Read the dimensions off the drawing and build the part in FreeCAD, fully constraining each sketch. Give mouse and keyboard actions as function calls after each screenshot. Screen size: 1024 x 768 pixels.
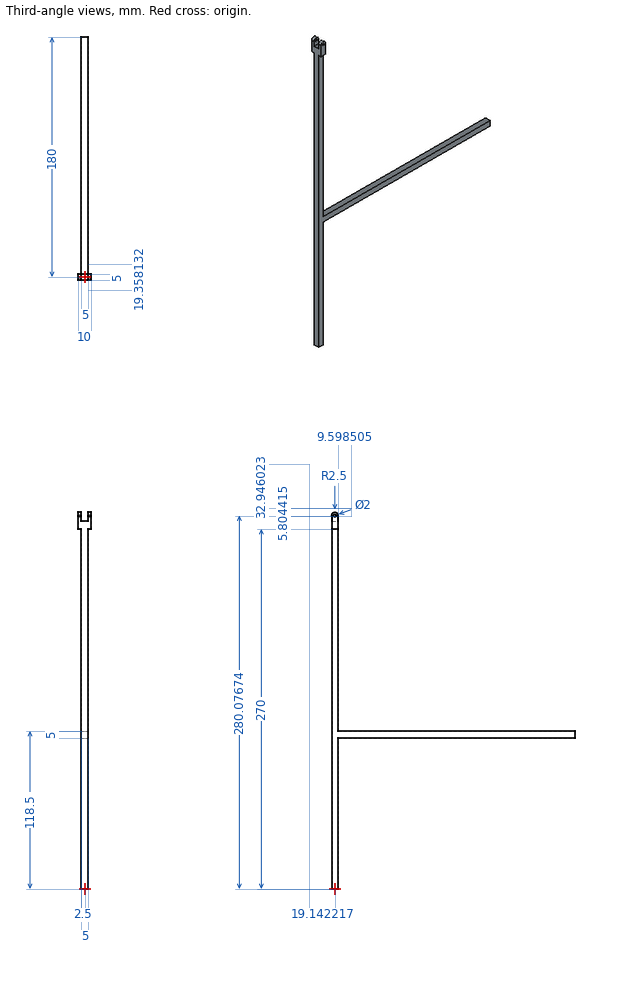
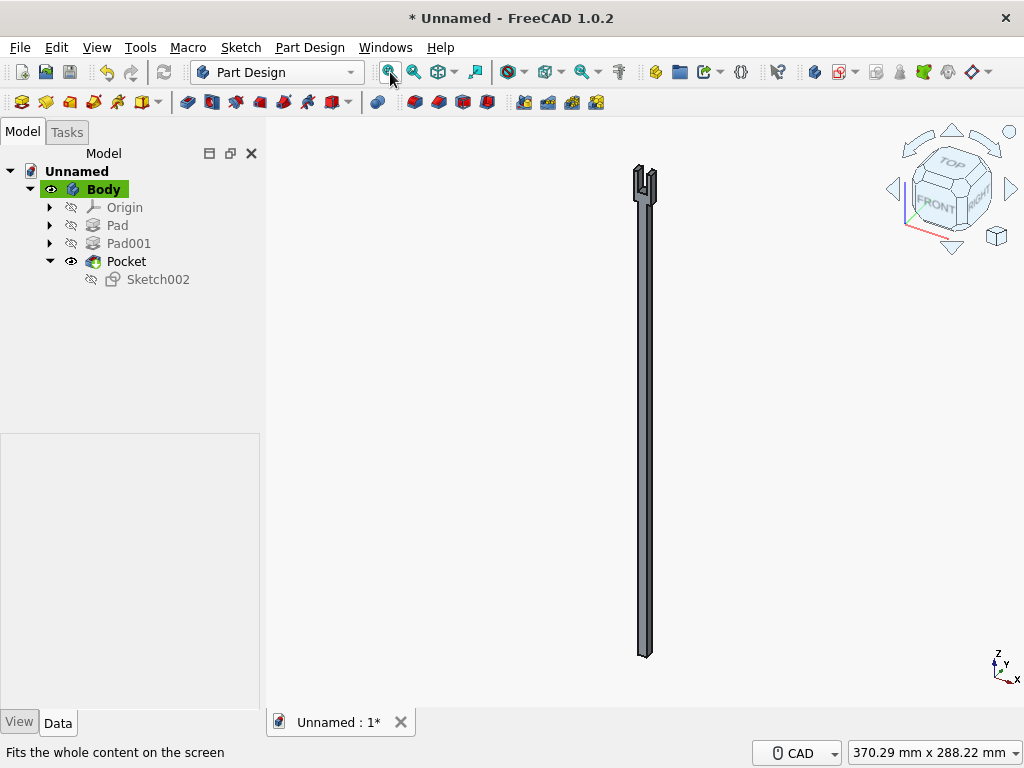
key(0)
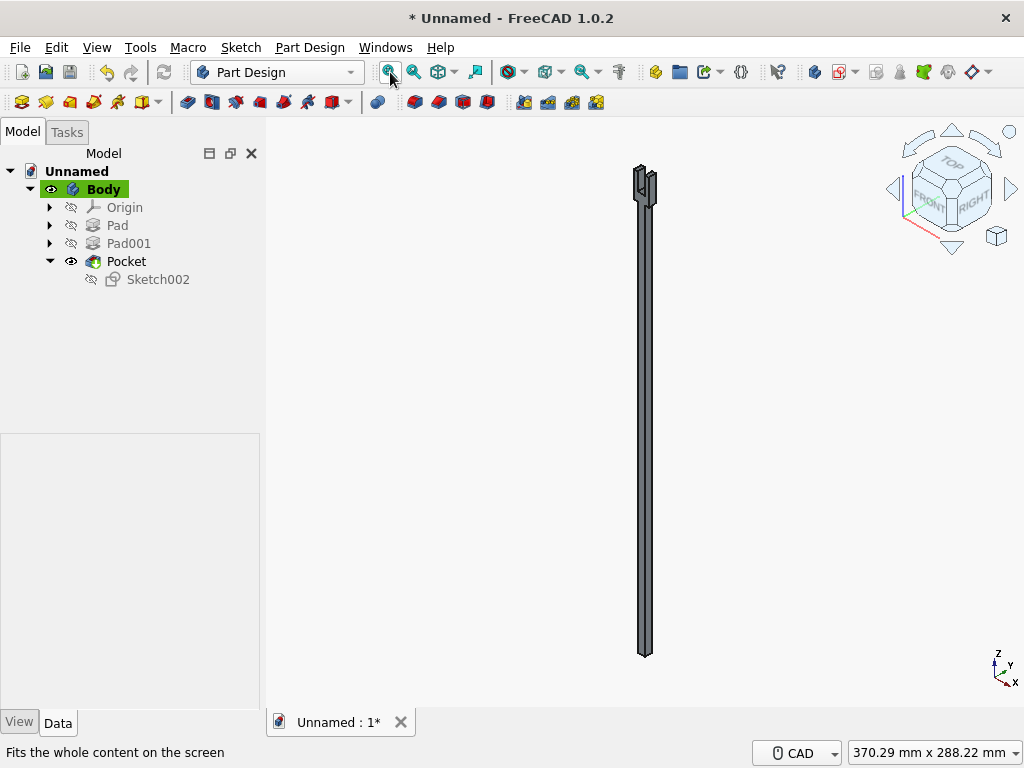
scroll(652, 181, up, 5)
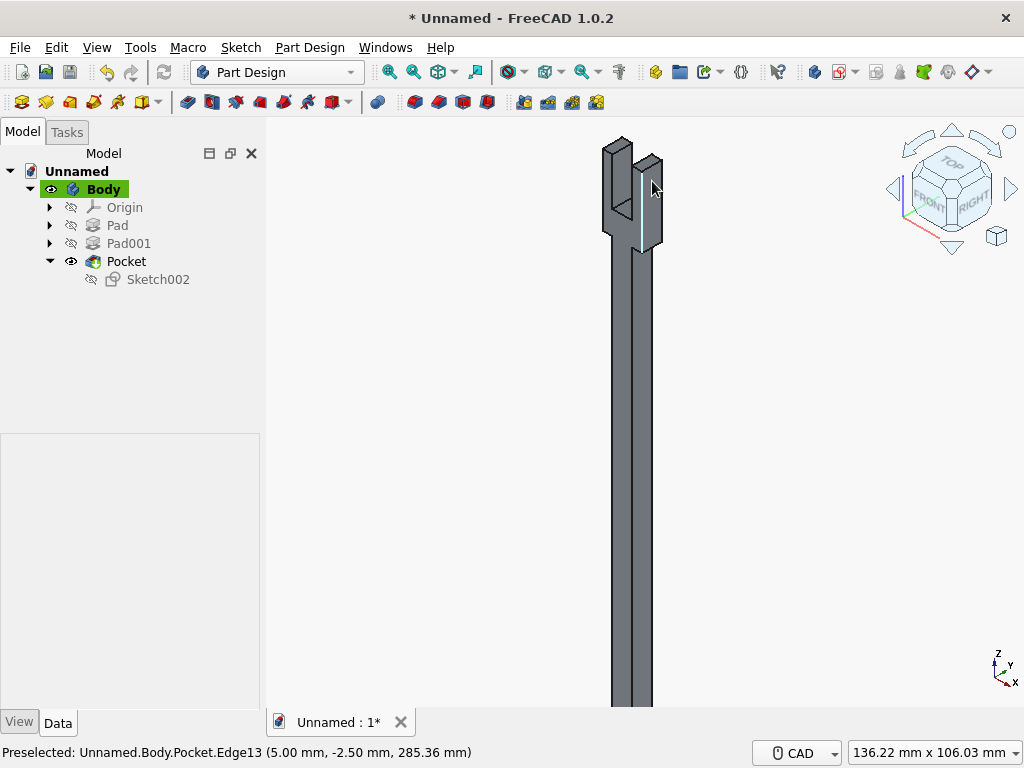
click(652, 182)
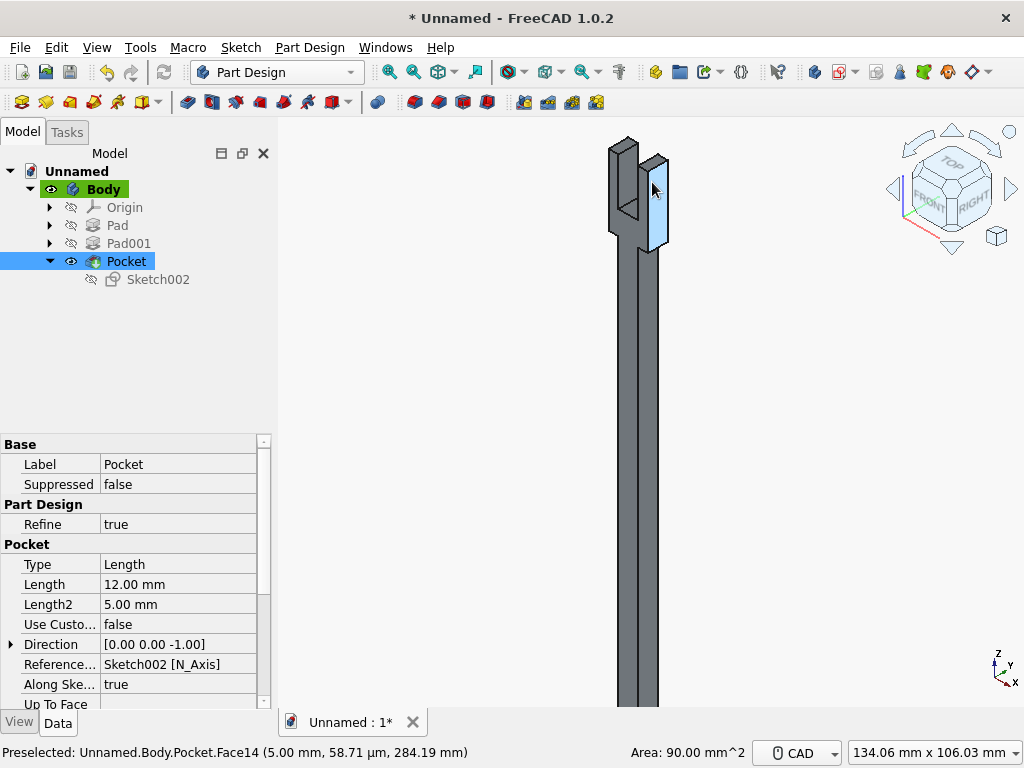
click(840, 72)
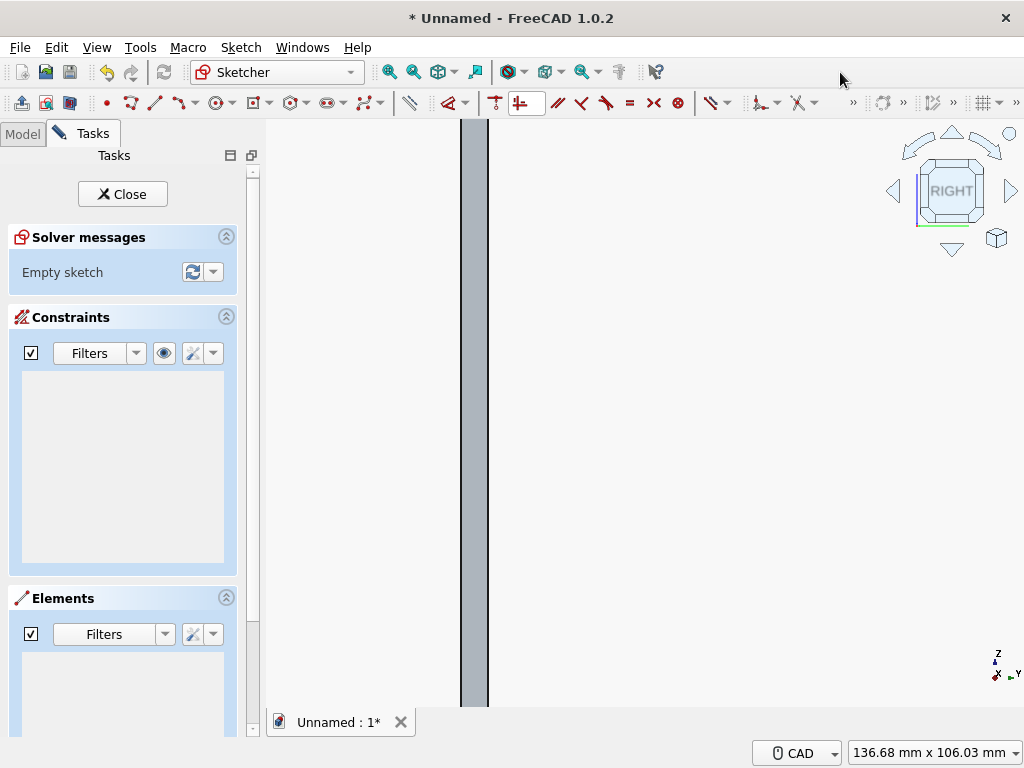
scroll(576, 413, down, 5)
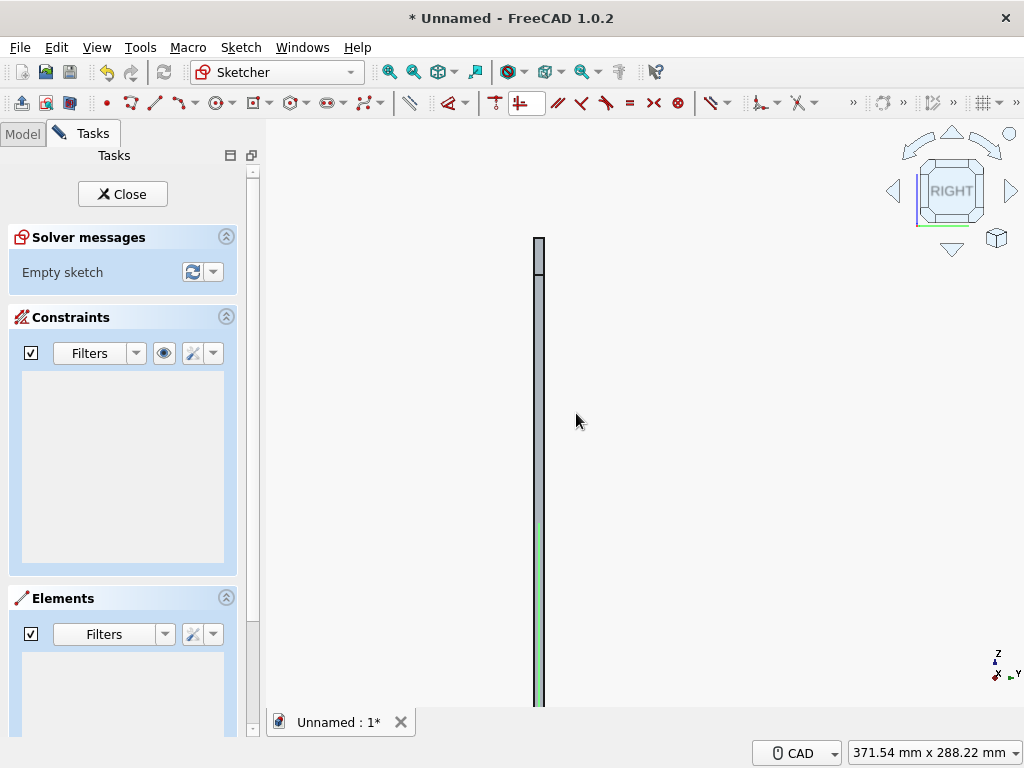
scroll(520, 166, up, 8)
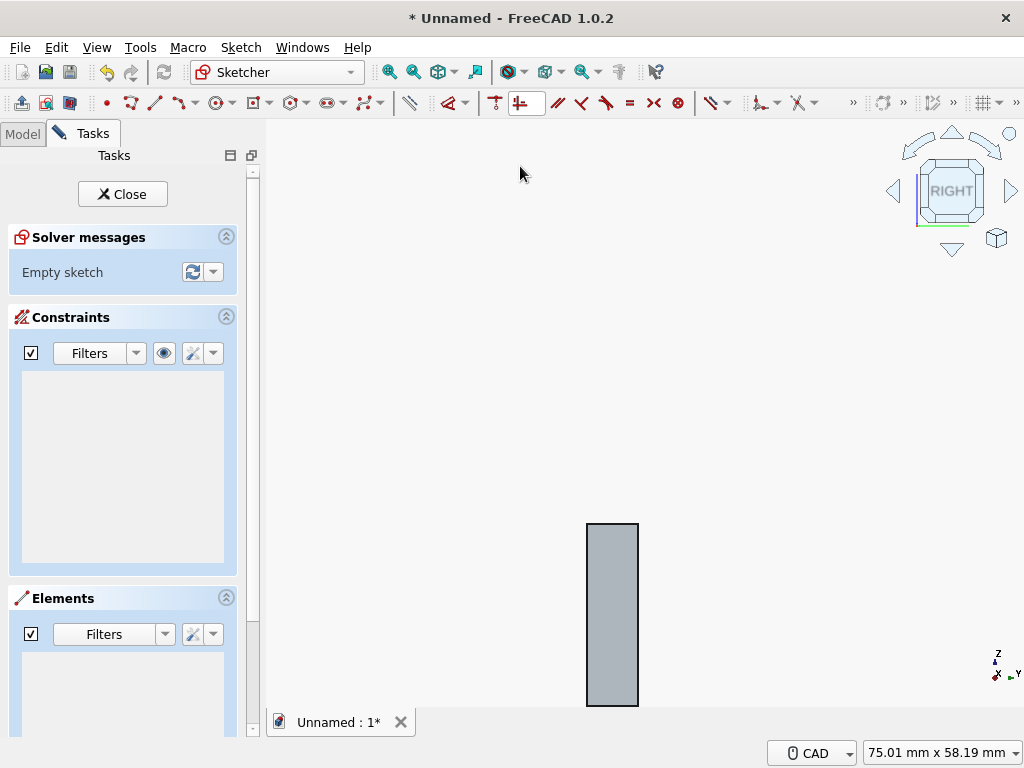
click(132, 104)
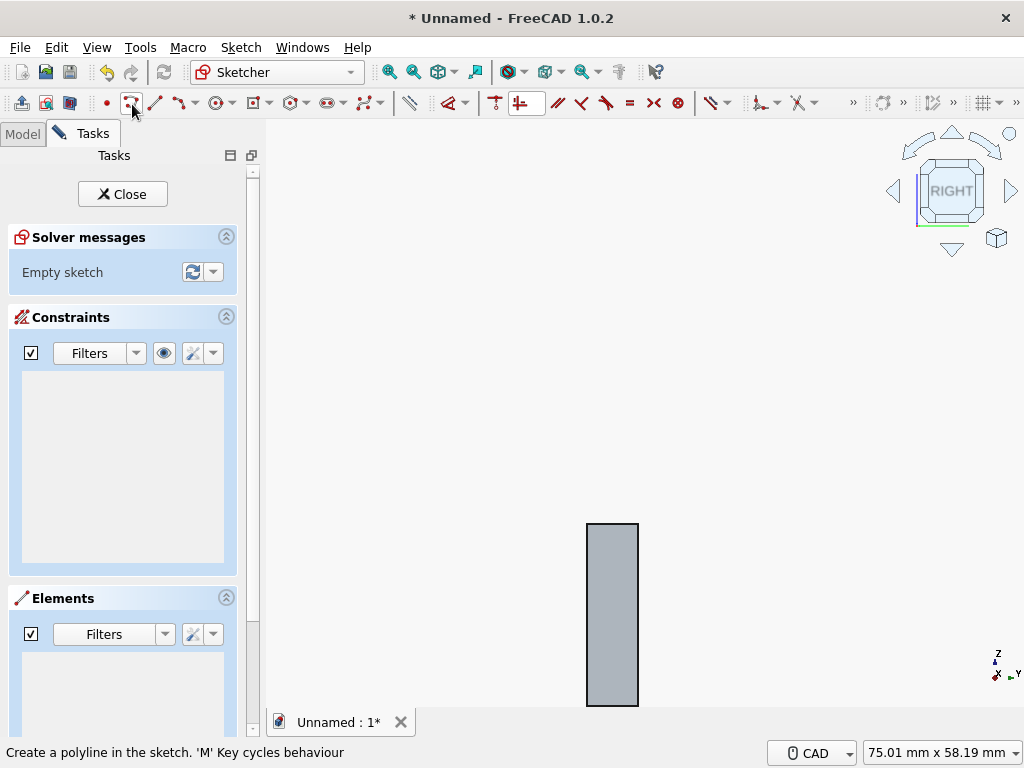
click(638, 604)
click(735, 604)
click(735, 545)
click(419, 212)
click(587, 604)
right_click(587, 604)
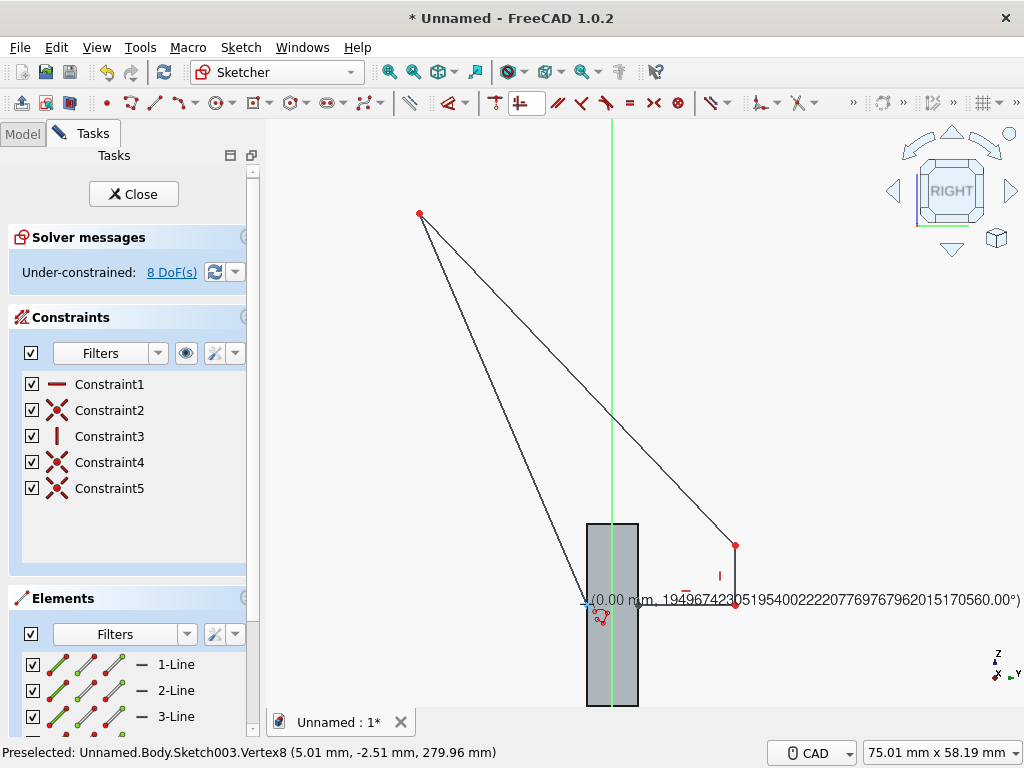
click(180, 104)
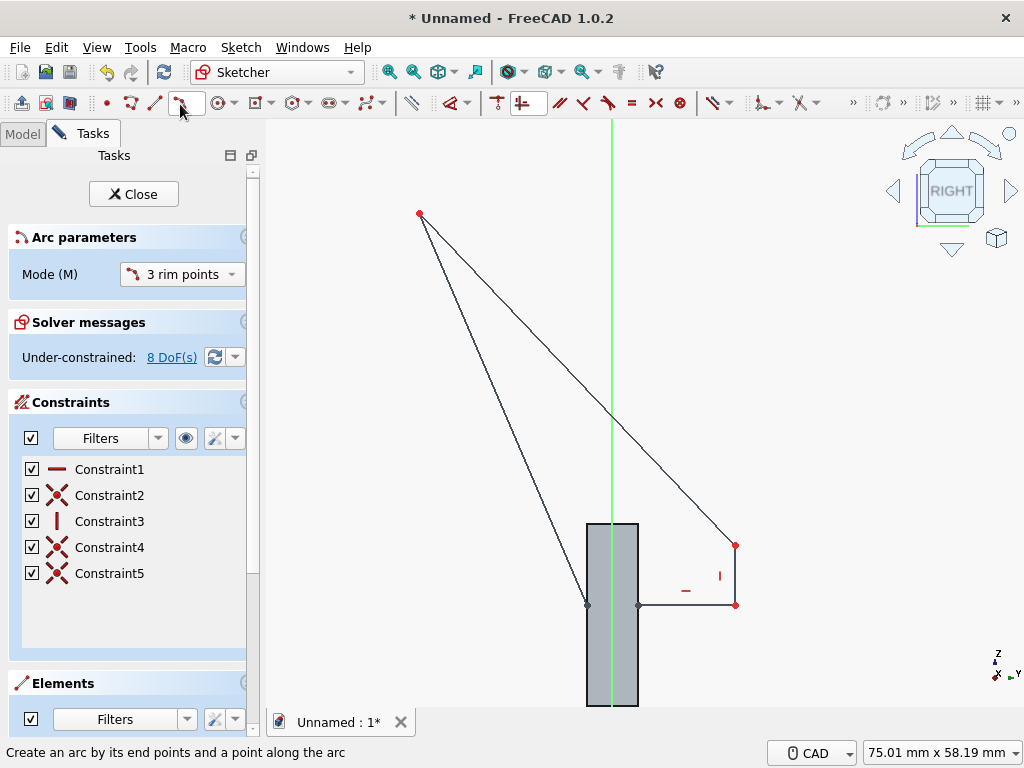
click(587, 605)
click(638, 605)
click(627, 583)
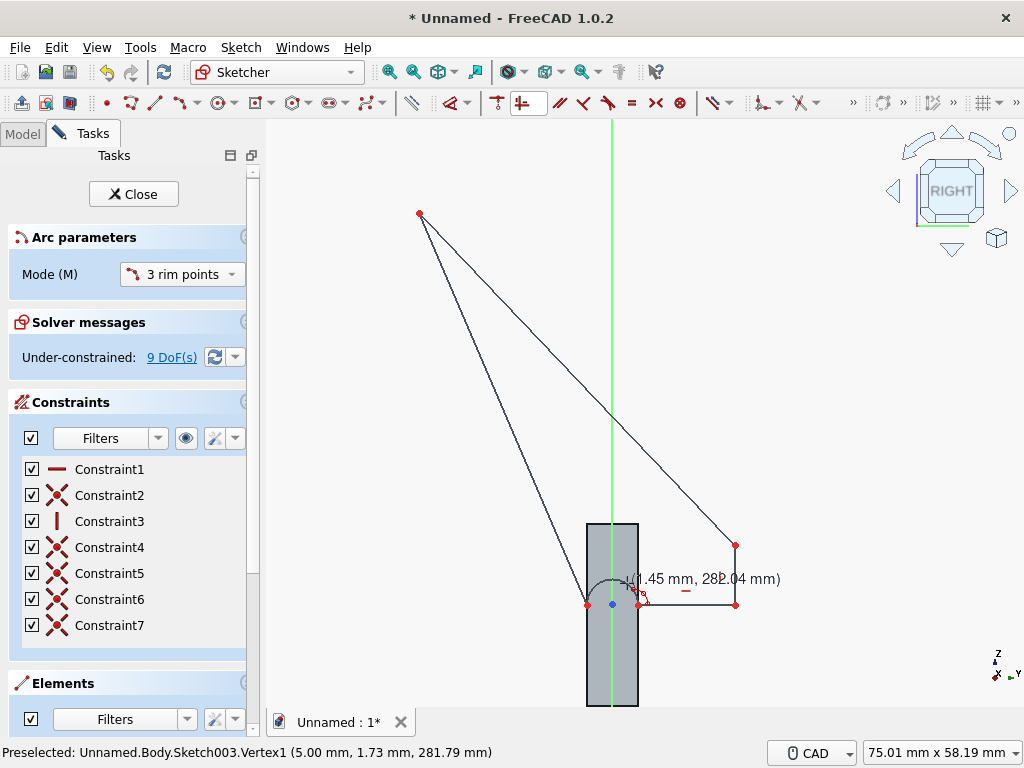
click(218, 104)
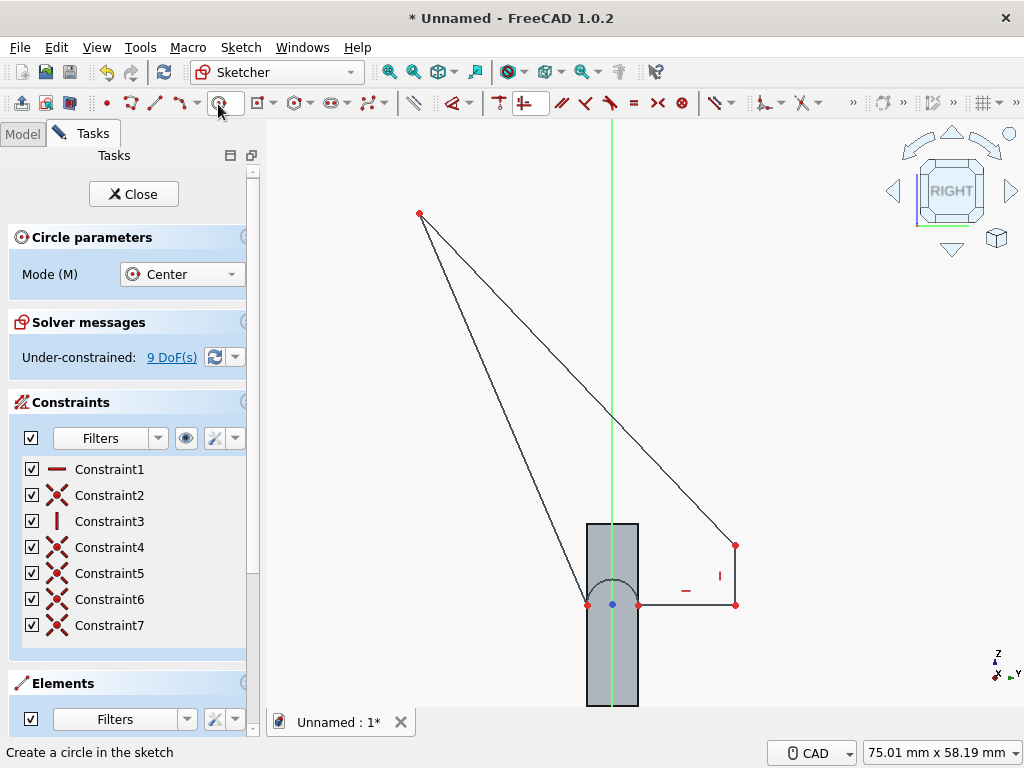
scroll(612, 604, up, 5)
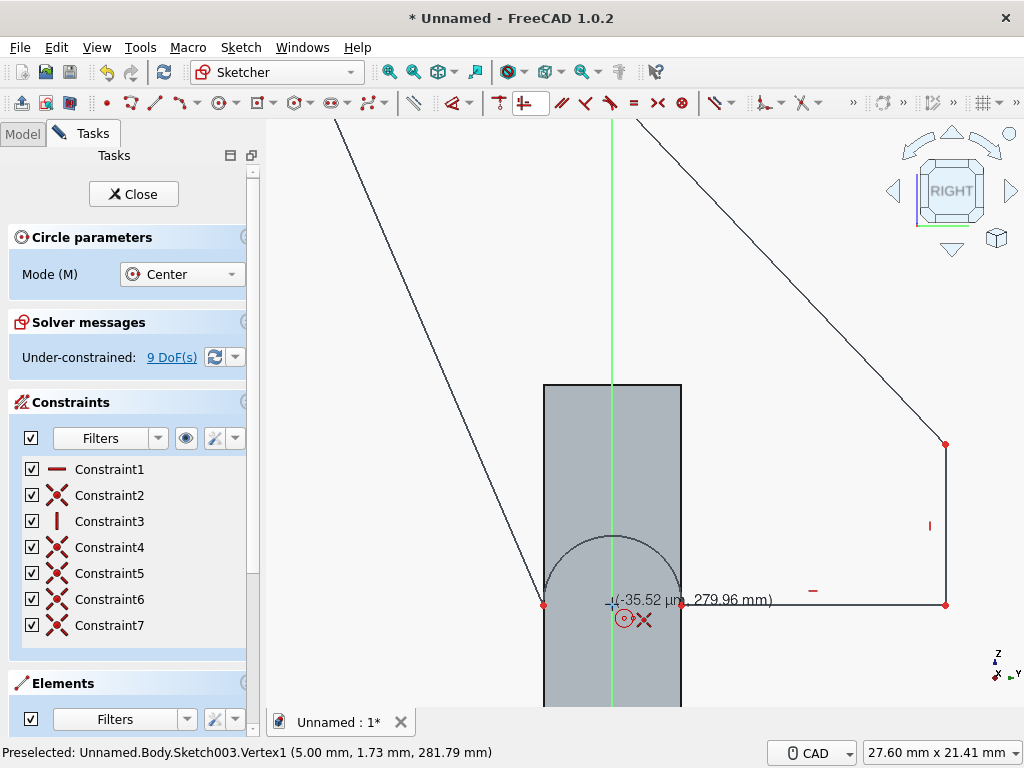
click(612, 602)
click(632, 583)
key(Escape)